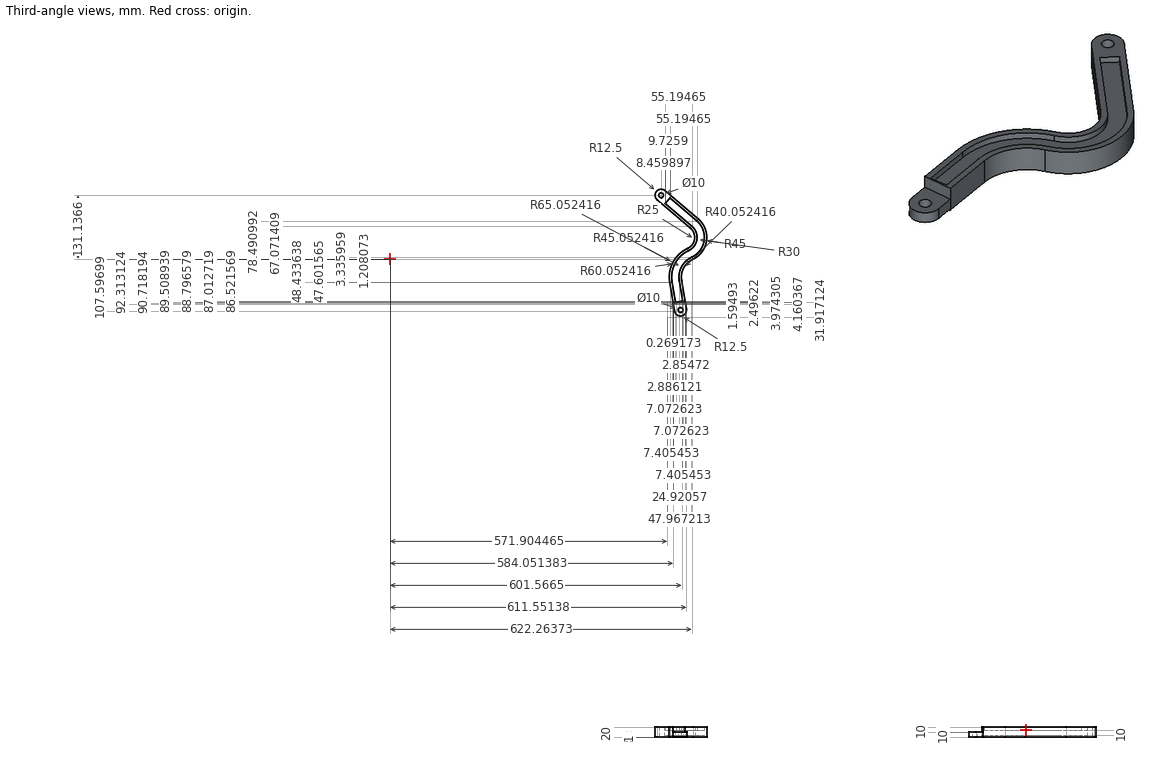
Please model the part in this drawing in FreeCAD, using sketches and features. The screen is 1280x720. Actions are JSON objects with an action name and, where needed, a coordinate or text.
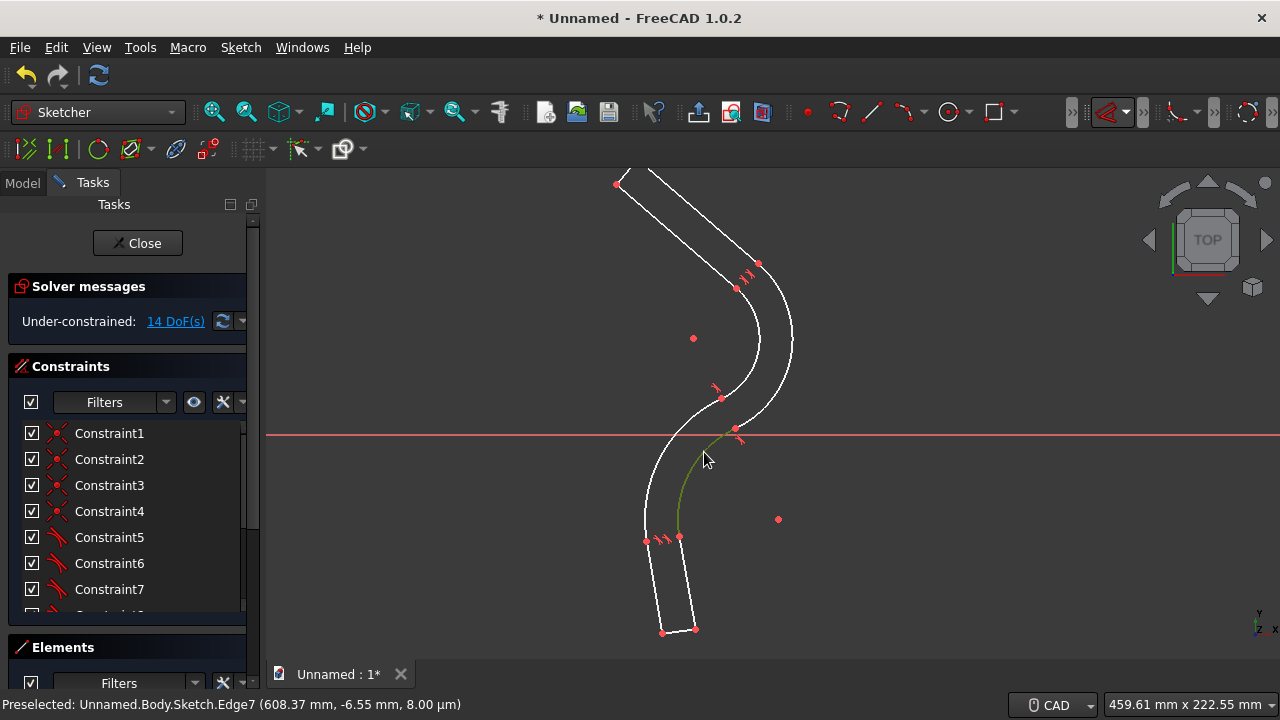
{"action": "key", "text": "k r"}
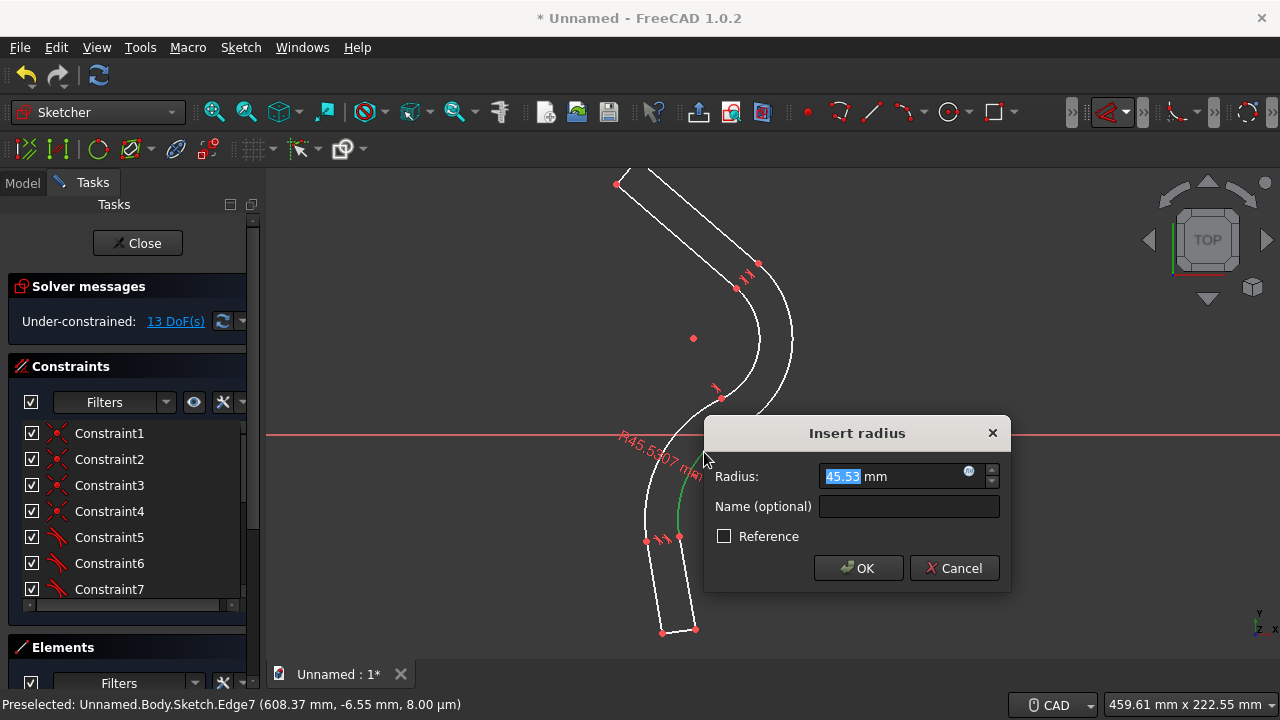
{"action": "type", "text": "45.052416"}
{"action": "key", "text": "Return"}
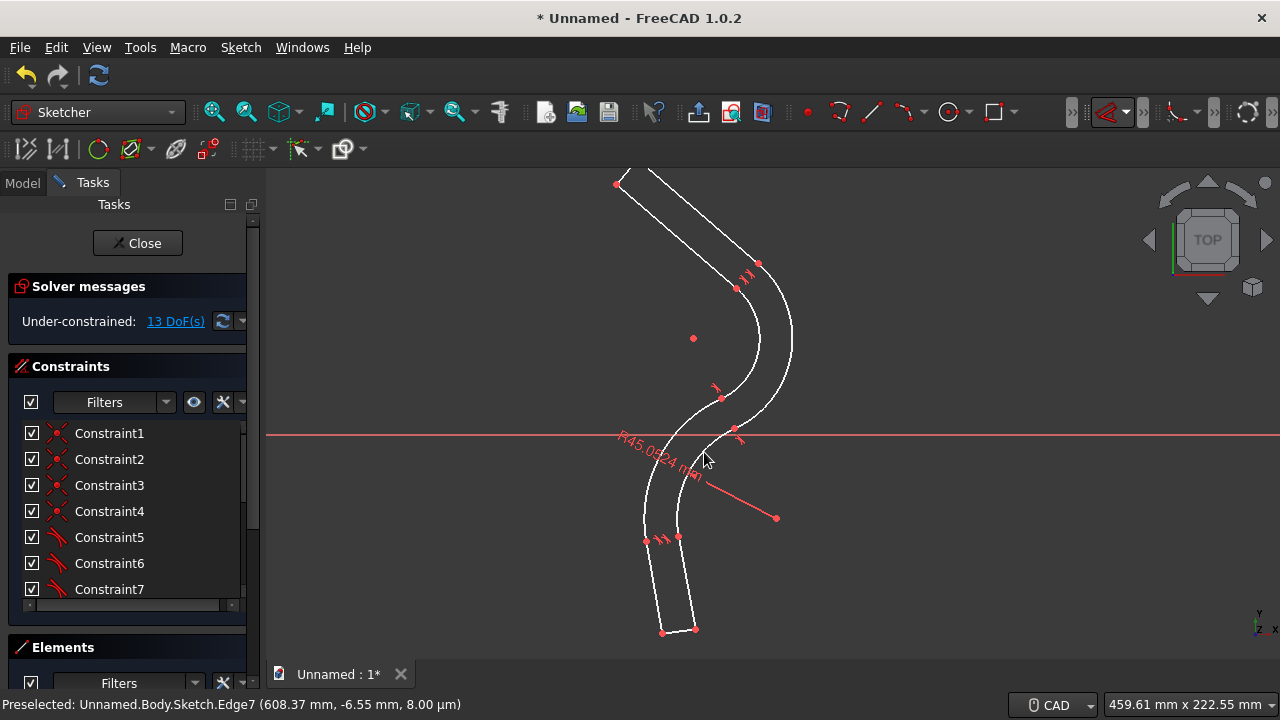
{"action": "left_click", "coordinate": [778, 390]}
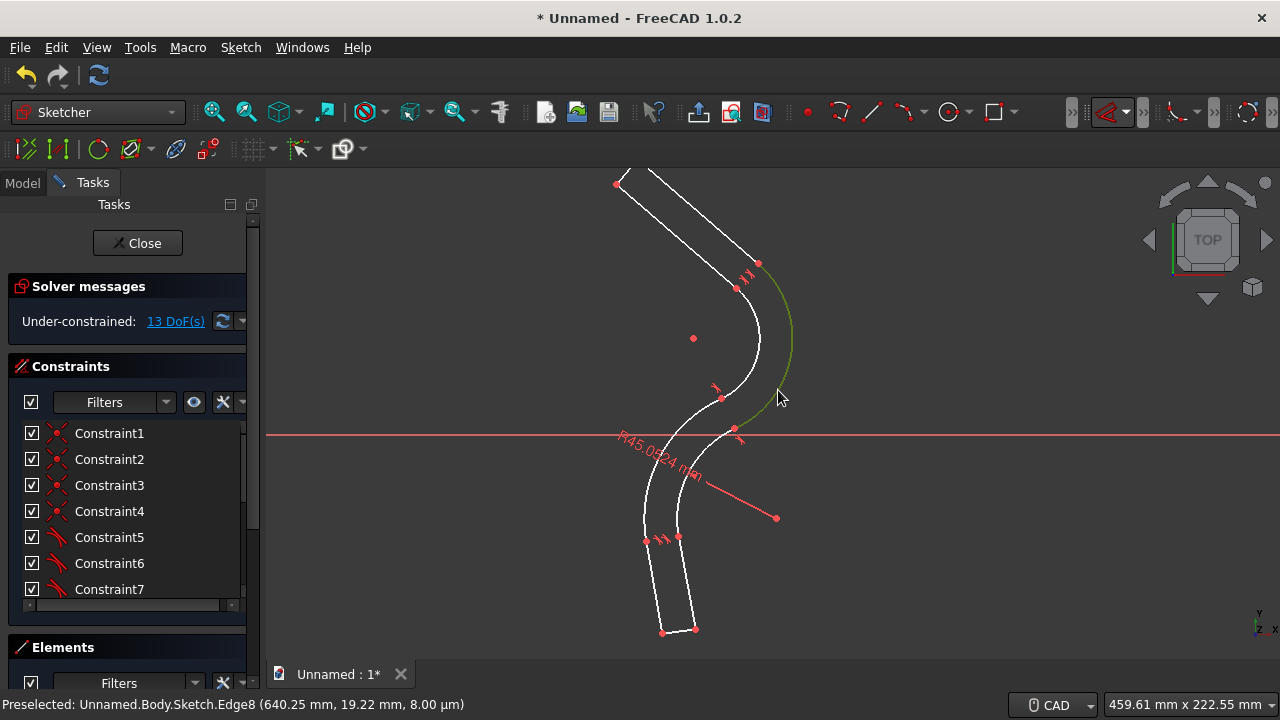
{"action": "key", "text": "k r"}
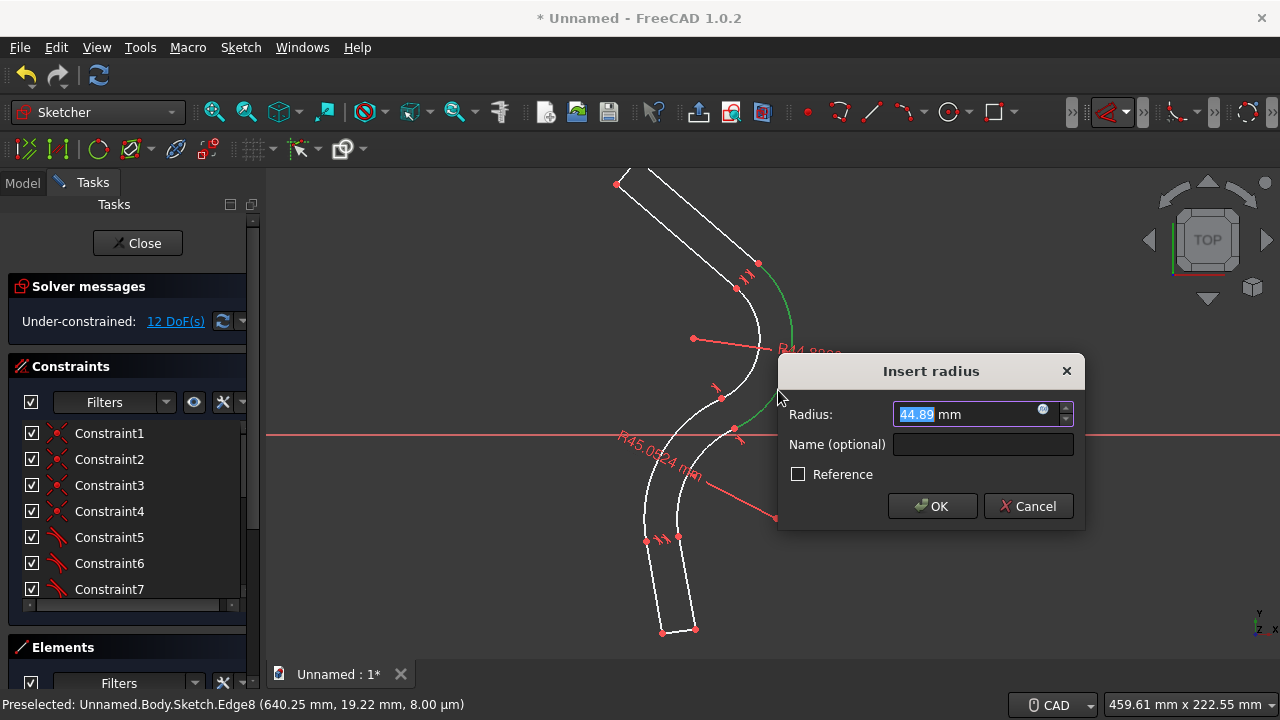
{"action": "type", "text": "45"}
{"action": "key", "text": "Return"}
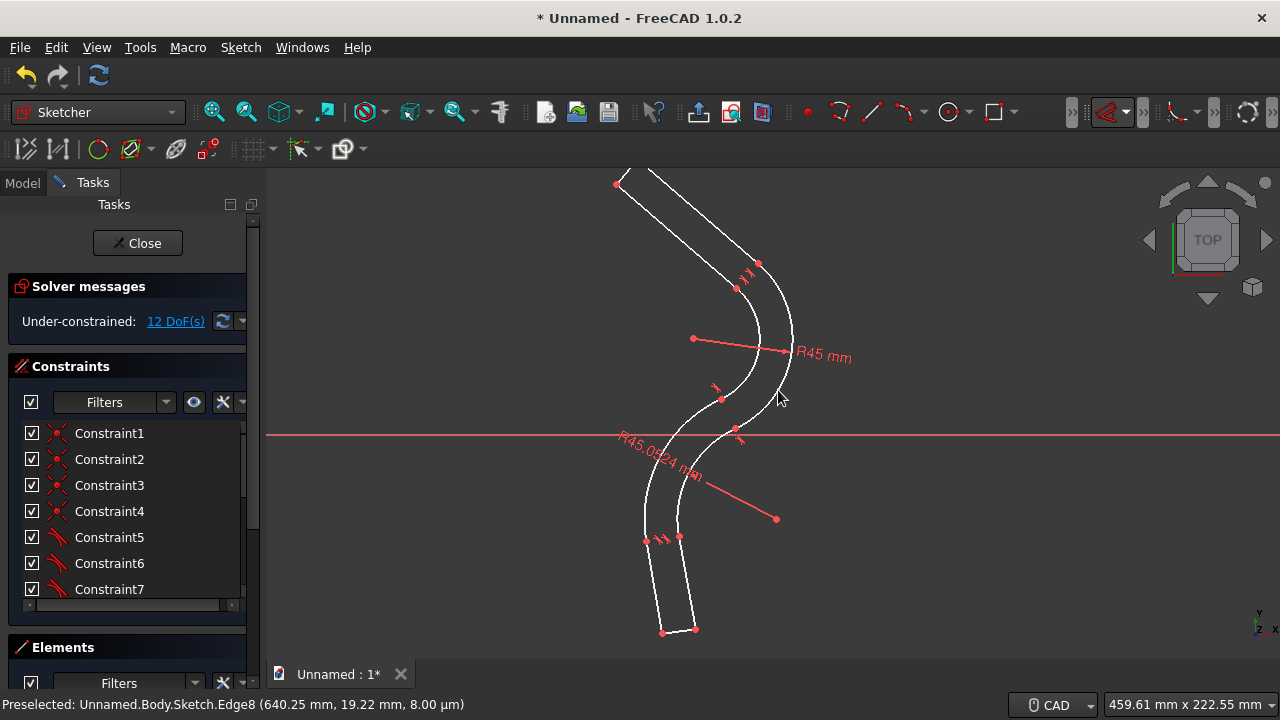
{"action": "left_click", "coordinate": [750, 373]}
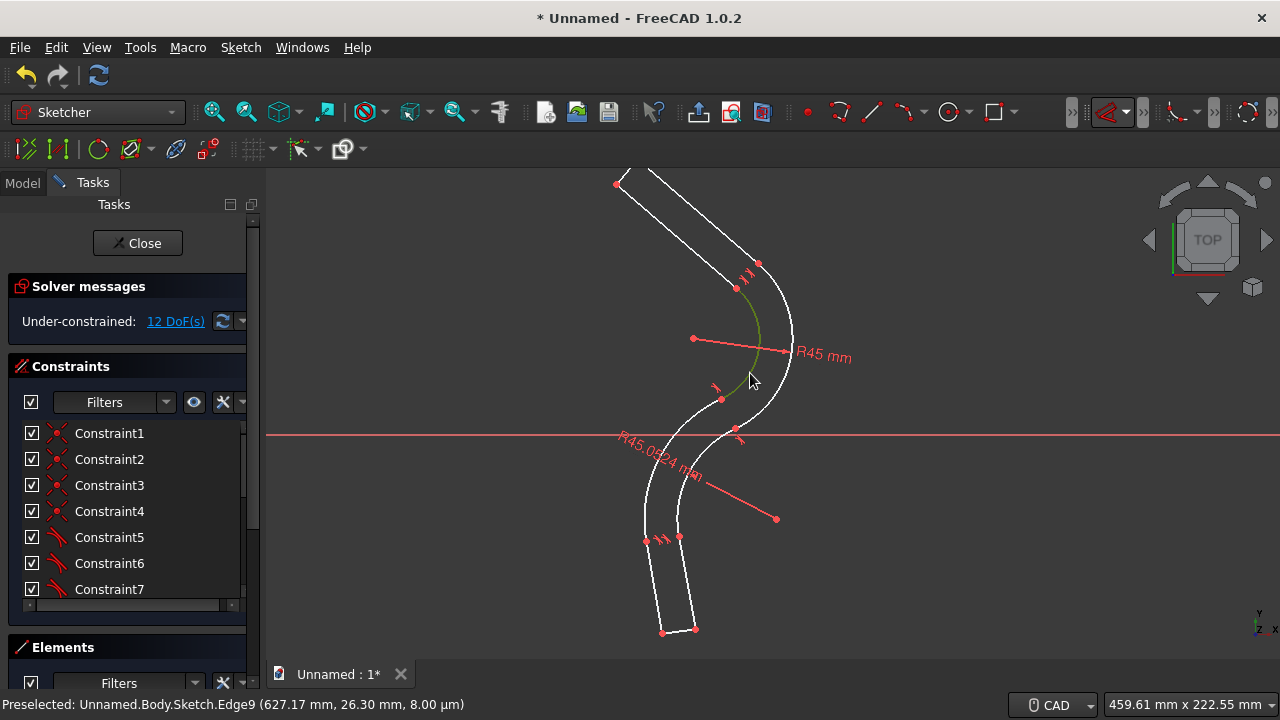
{"action": "left_click", "coordinate": [1128, 112]}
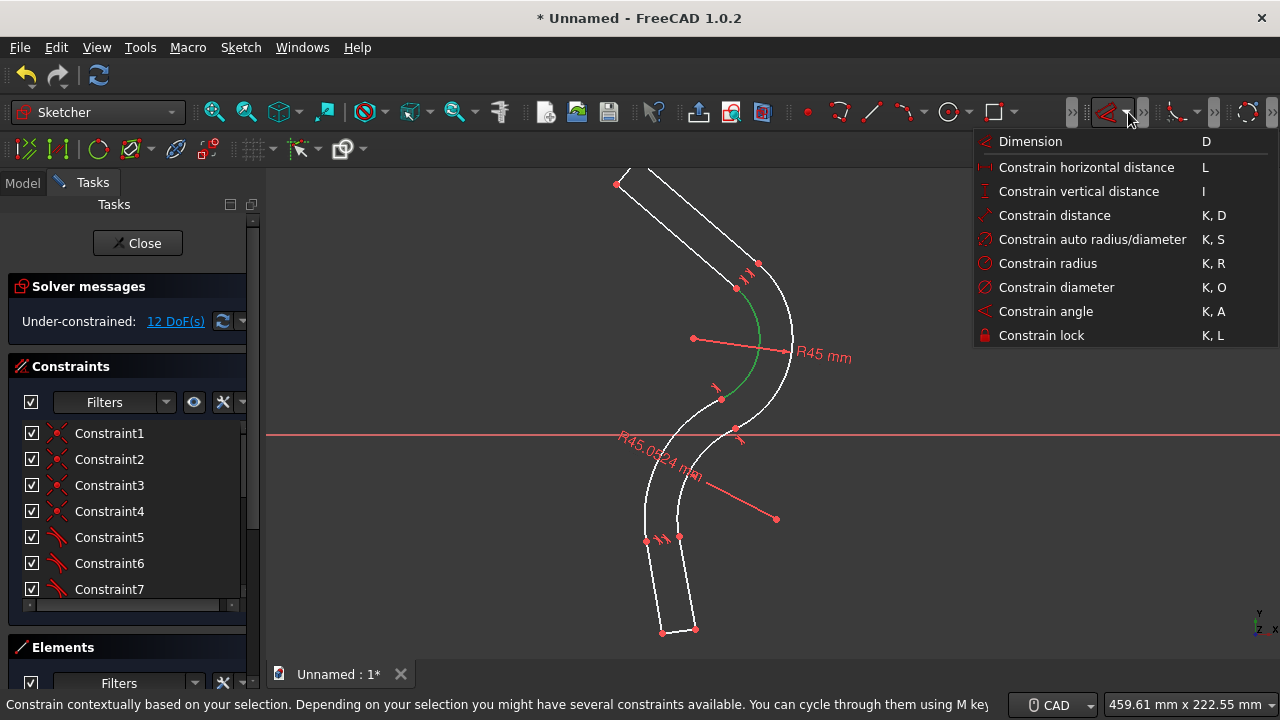
{"action": "left_click", "coordinate": [1126, 263]}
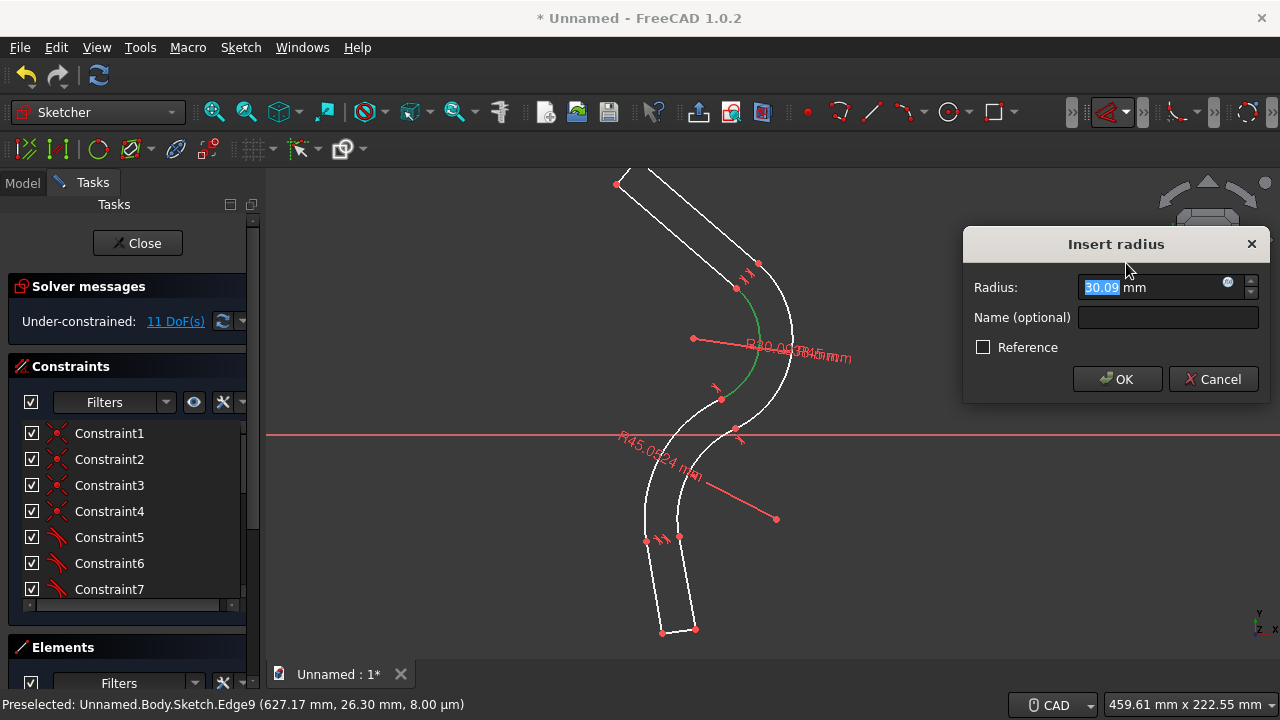
{"action": "type", "text": "30"}
{"action": "key", "text": "Return"}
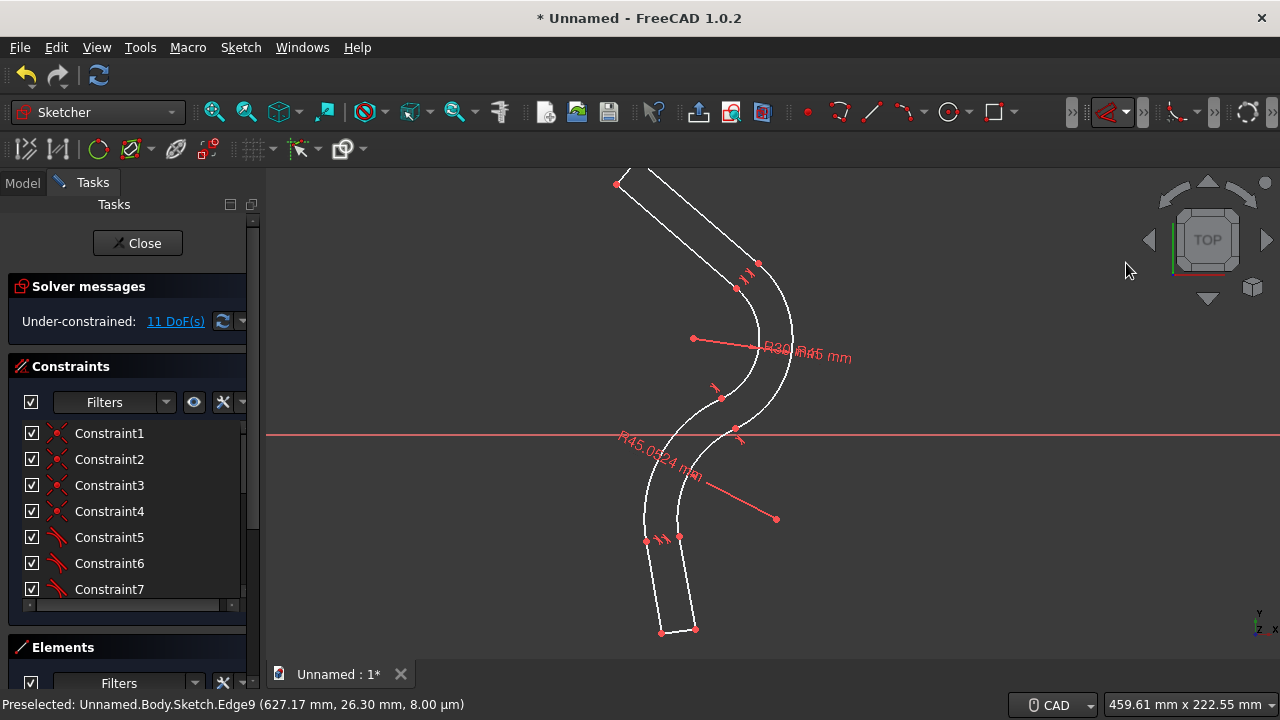
{"action": "scroll", "coordinate": [704, 450], "scroll_direction": "down", "scroll_amount": 2}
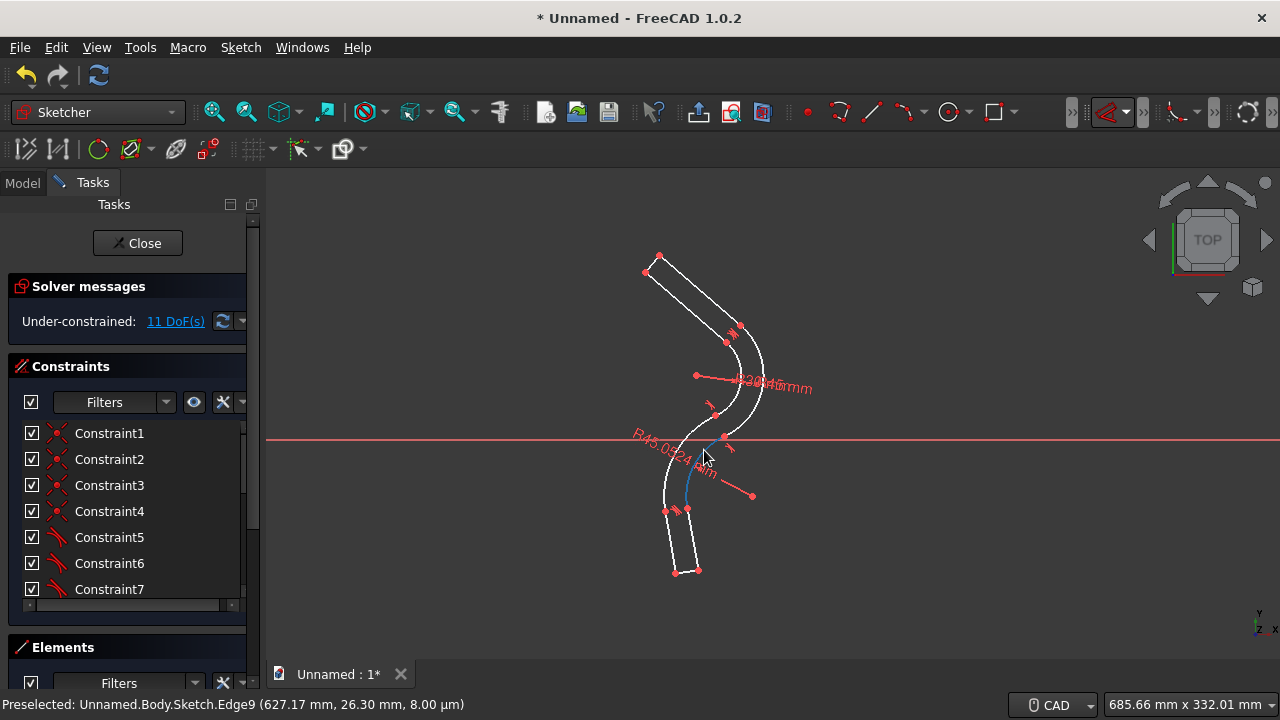
{"action": "scroll", "coordinate": [655, 260], "scroll_direction": "up", "scroll_amount": 6}